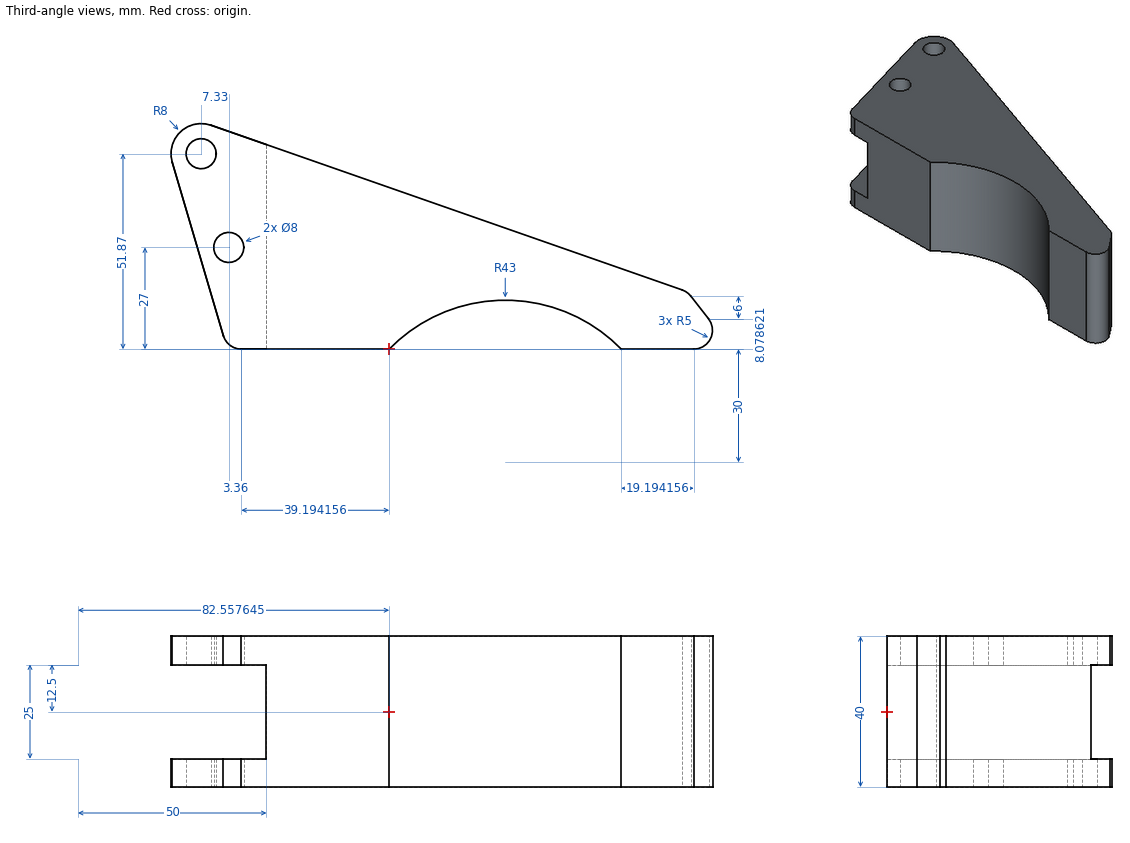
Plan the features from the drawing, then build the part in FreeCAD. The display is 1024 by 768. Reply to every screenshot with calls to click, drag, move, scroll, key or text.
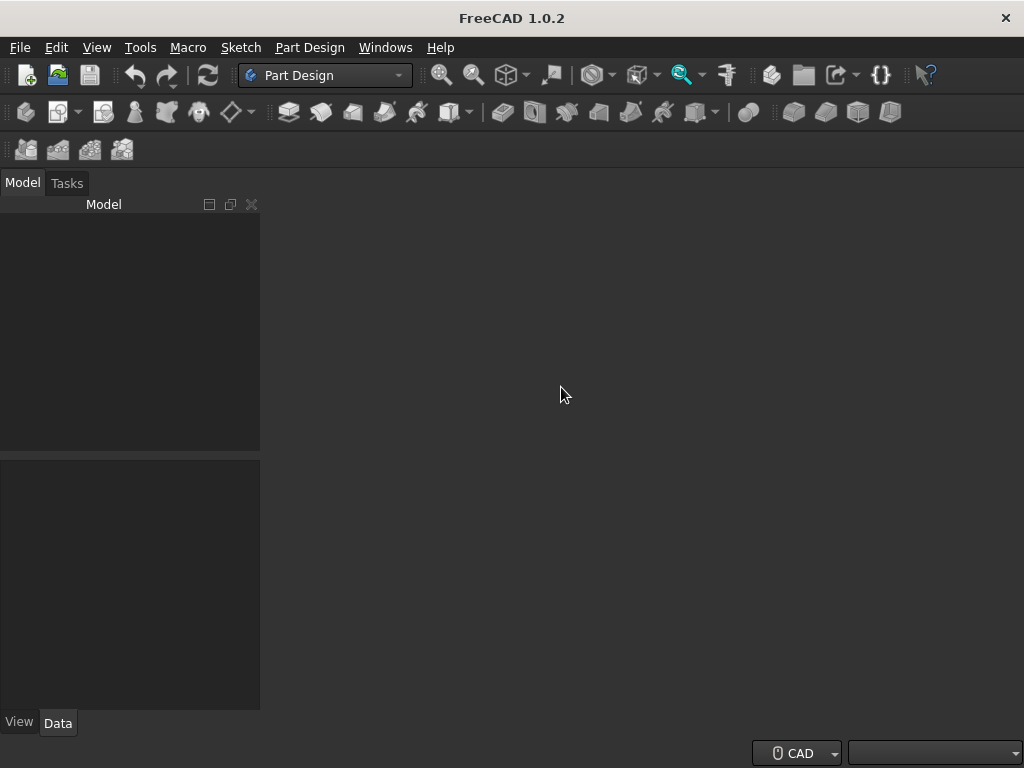
click(26, 76)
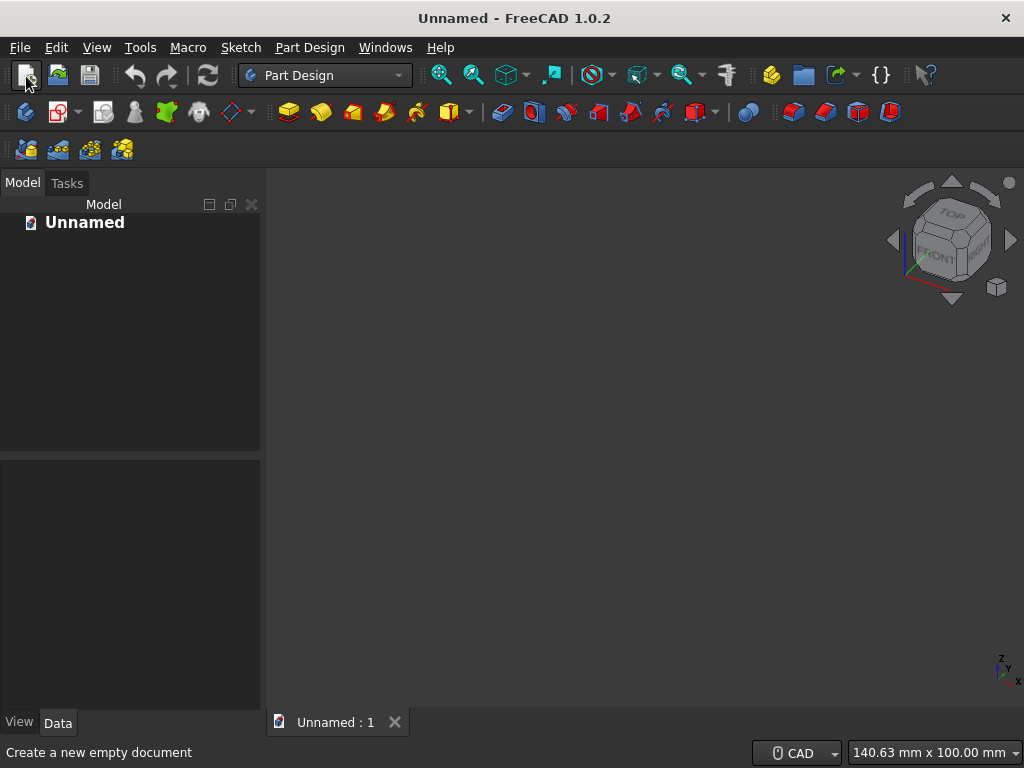
click(58, 112)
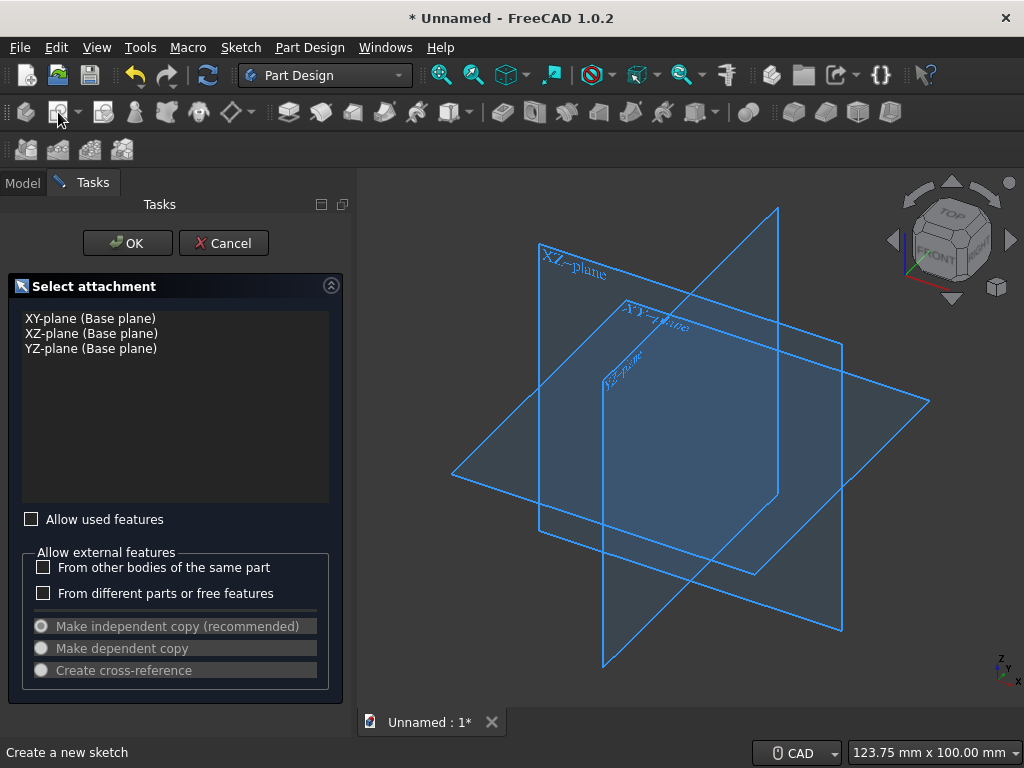
click(82, 318)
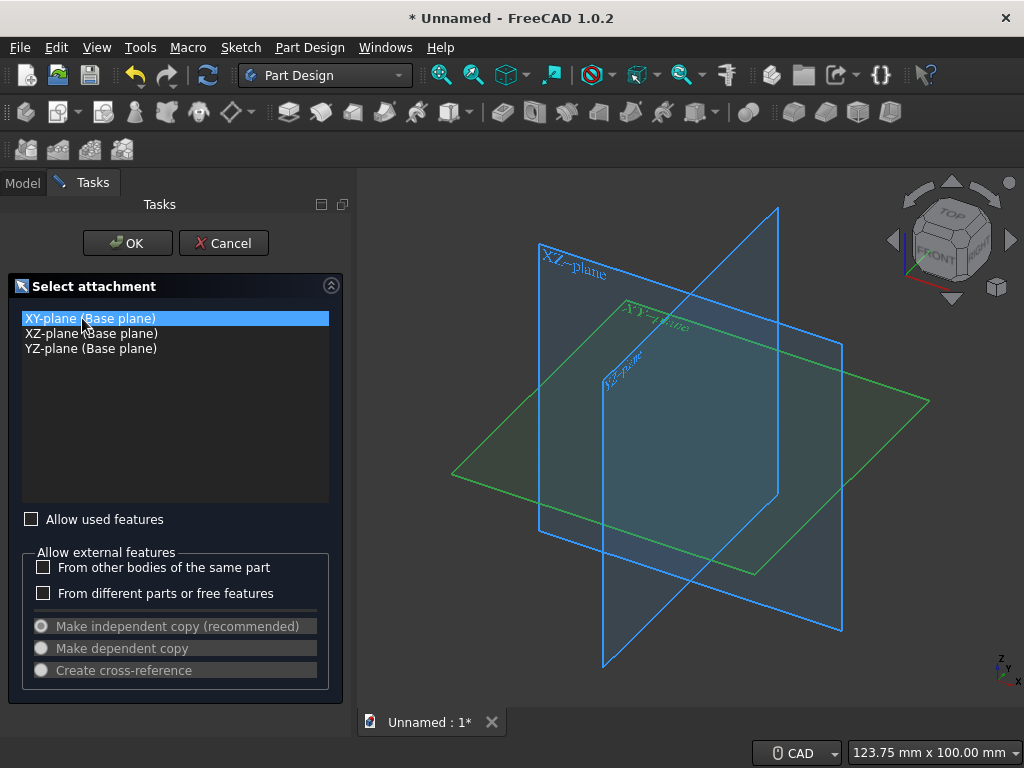
click(128, 243)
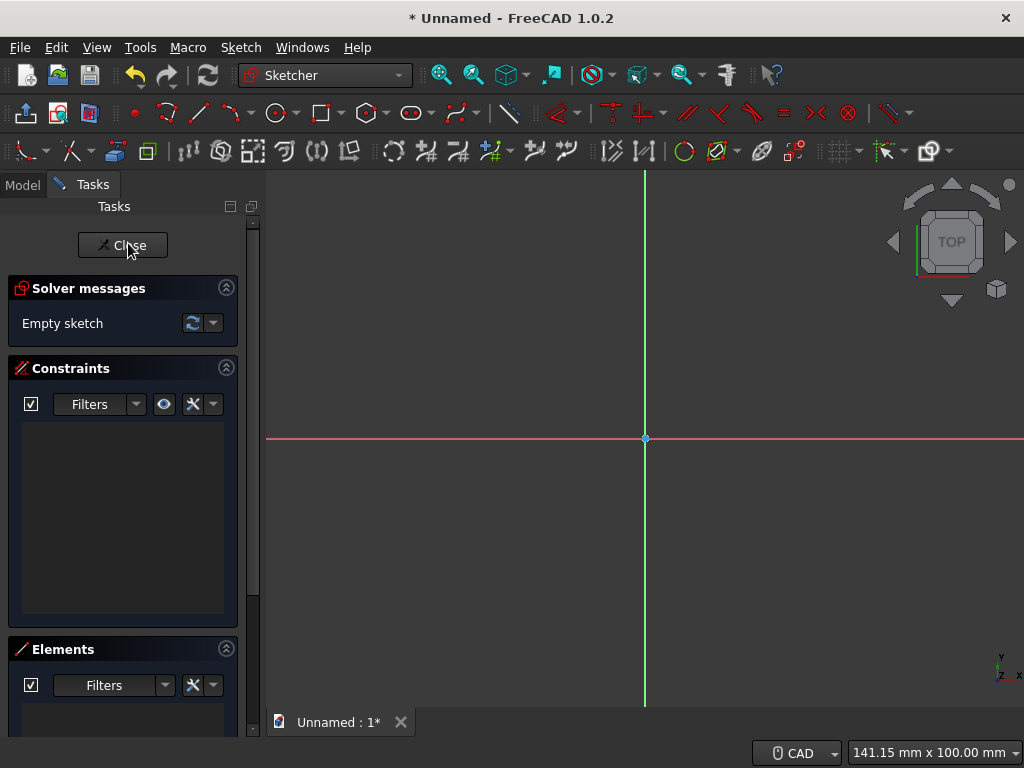
scroll(403, 633, down, 3)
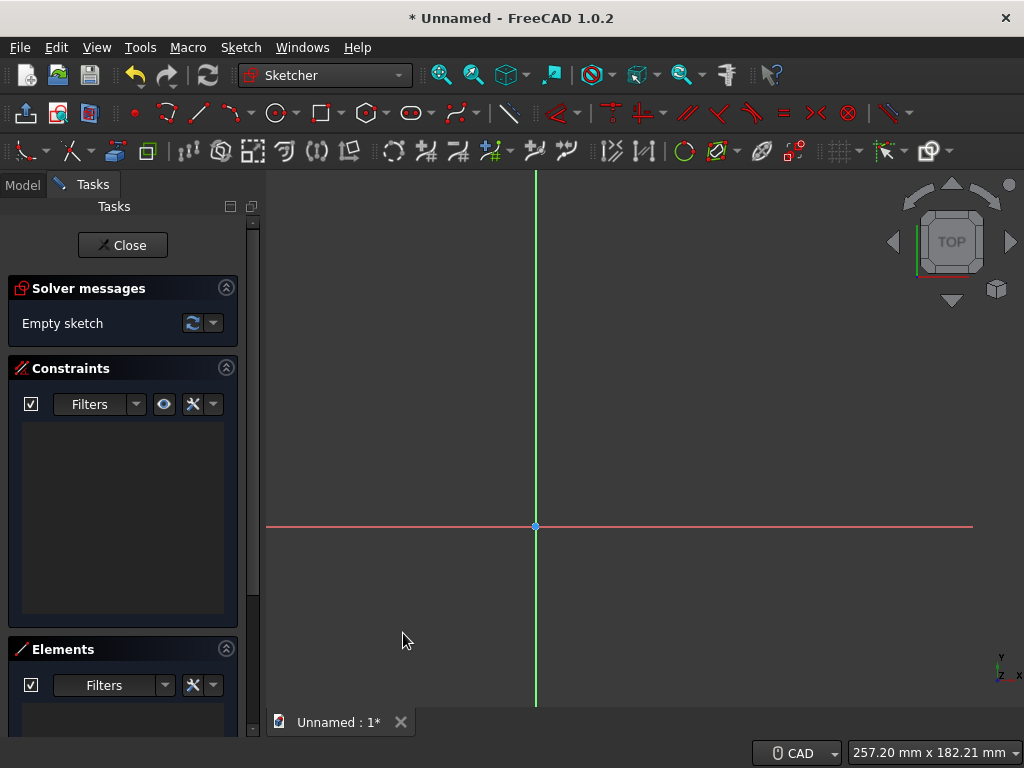
click(200, 114)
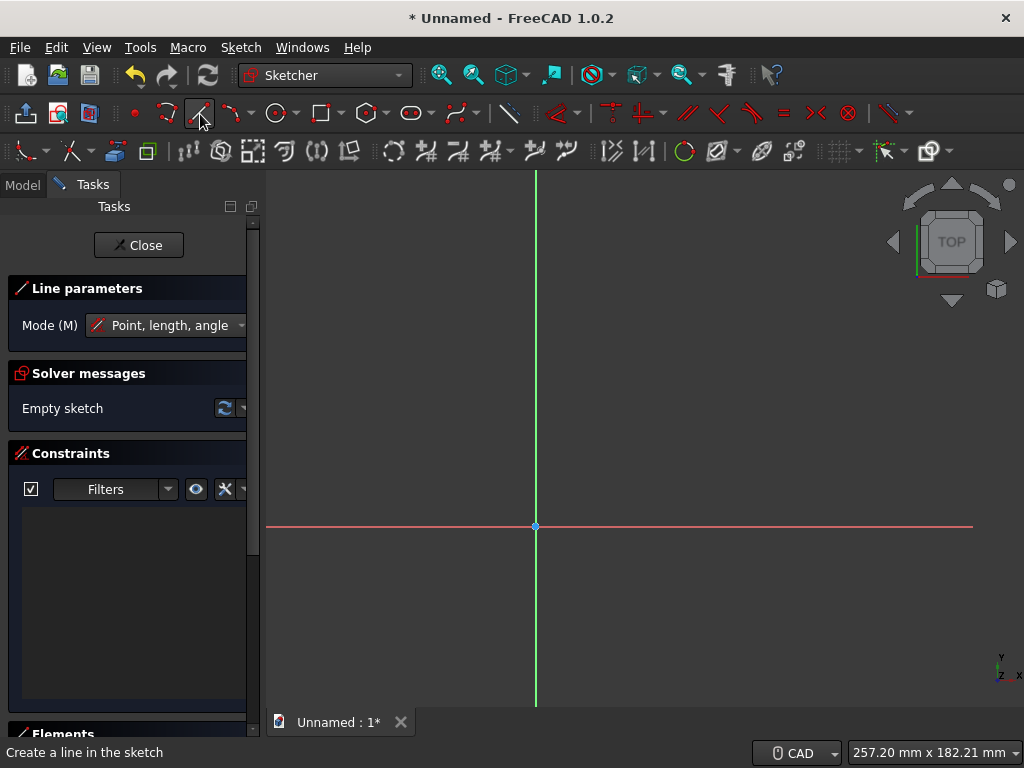
click(420, 527)
click(536, 527)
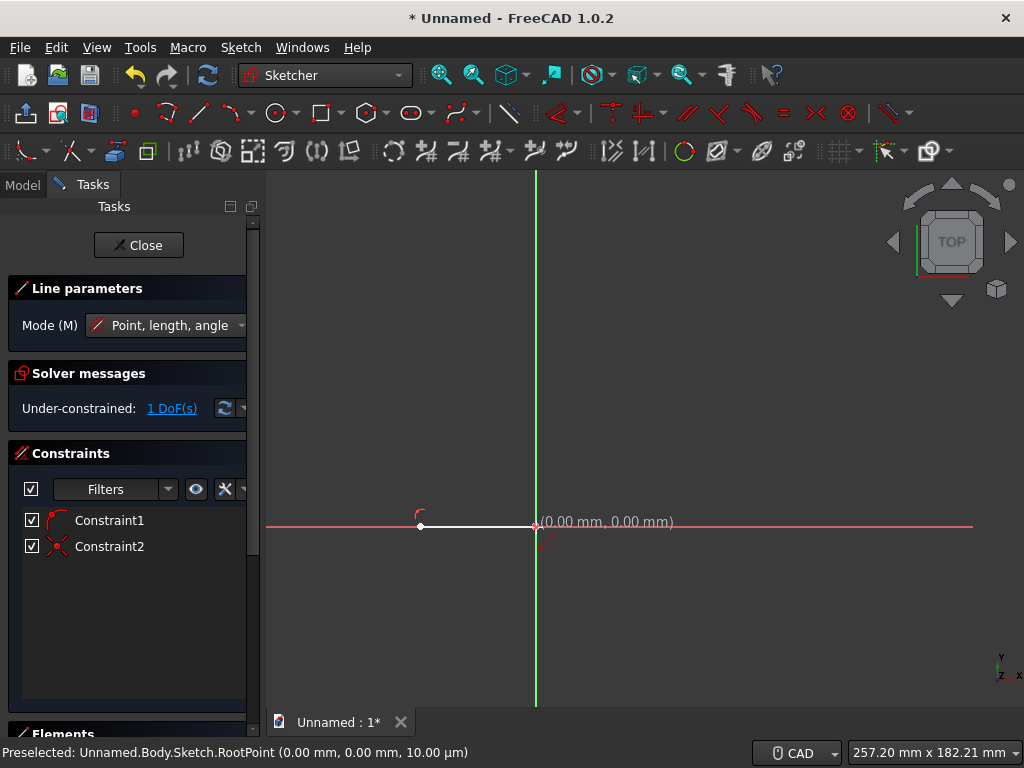
click(717, 527)
click(774, 518)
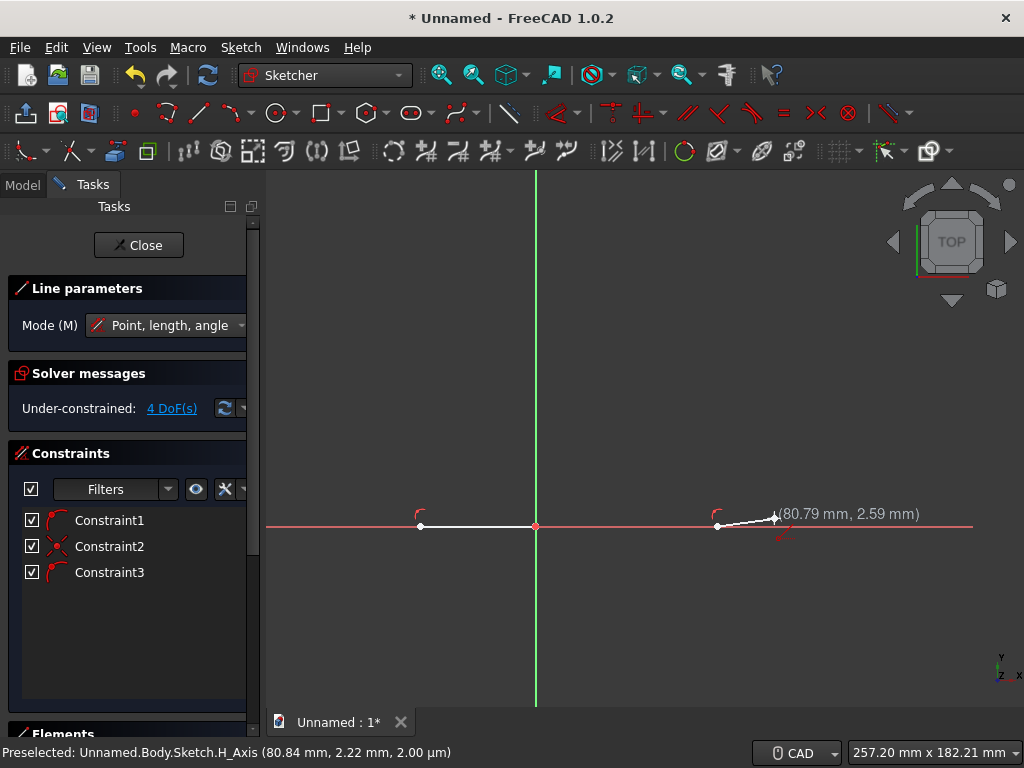
click(786, 503)
click(772, 485)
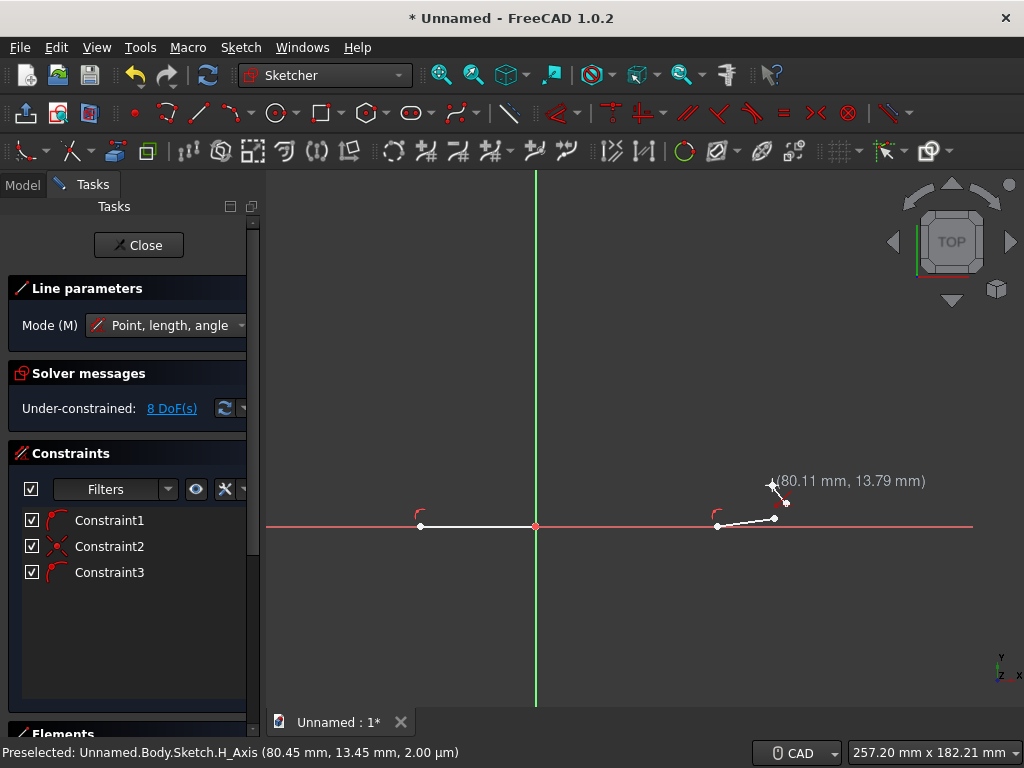
scroll(765, 480, up, 4)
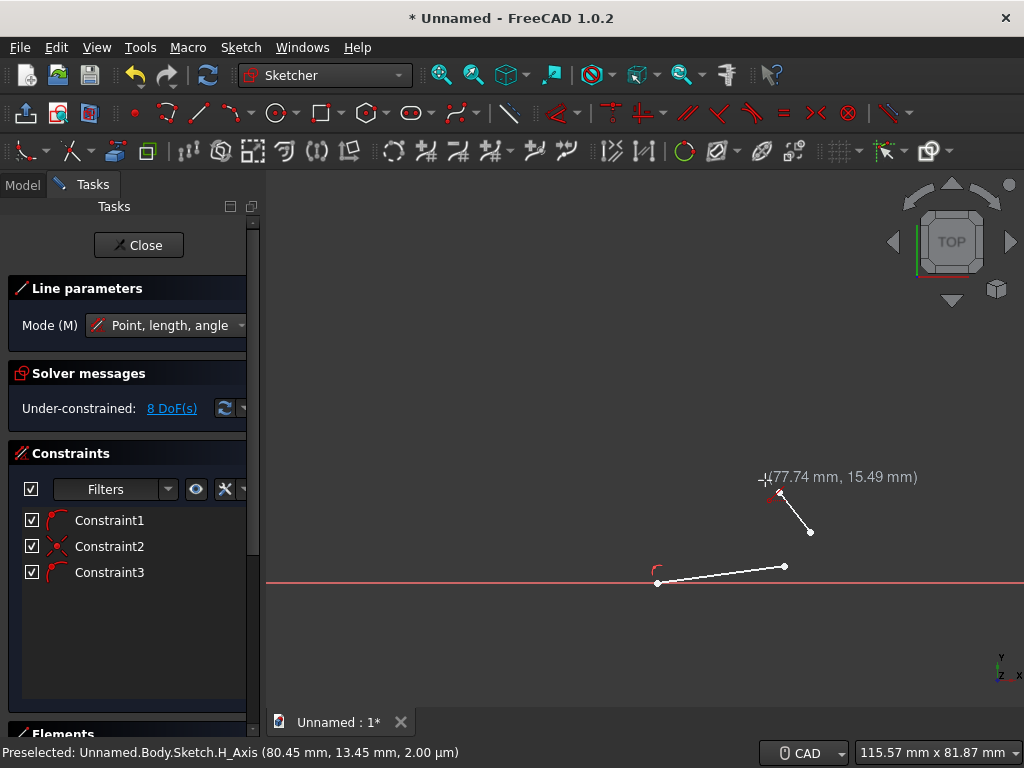
click(764, 480)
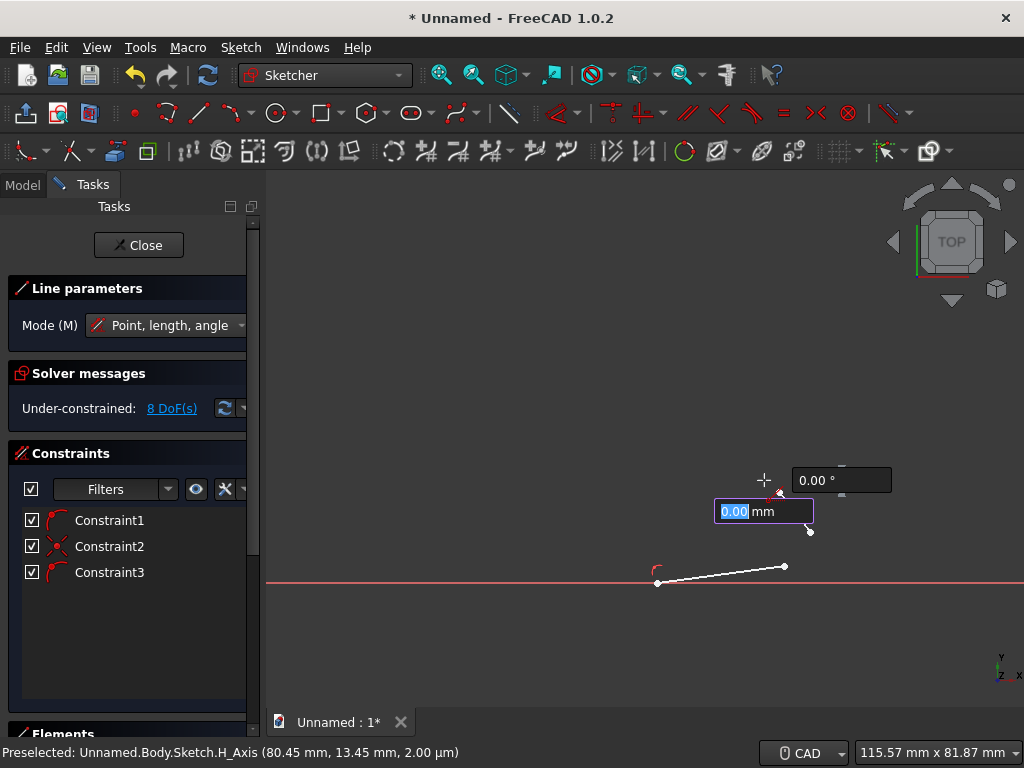
scroll(765, 480, down, 4)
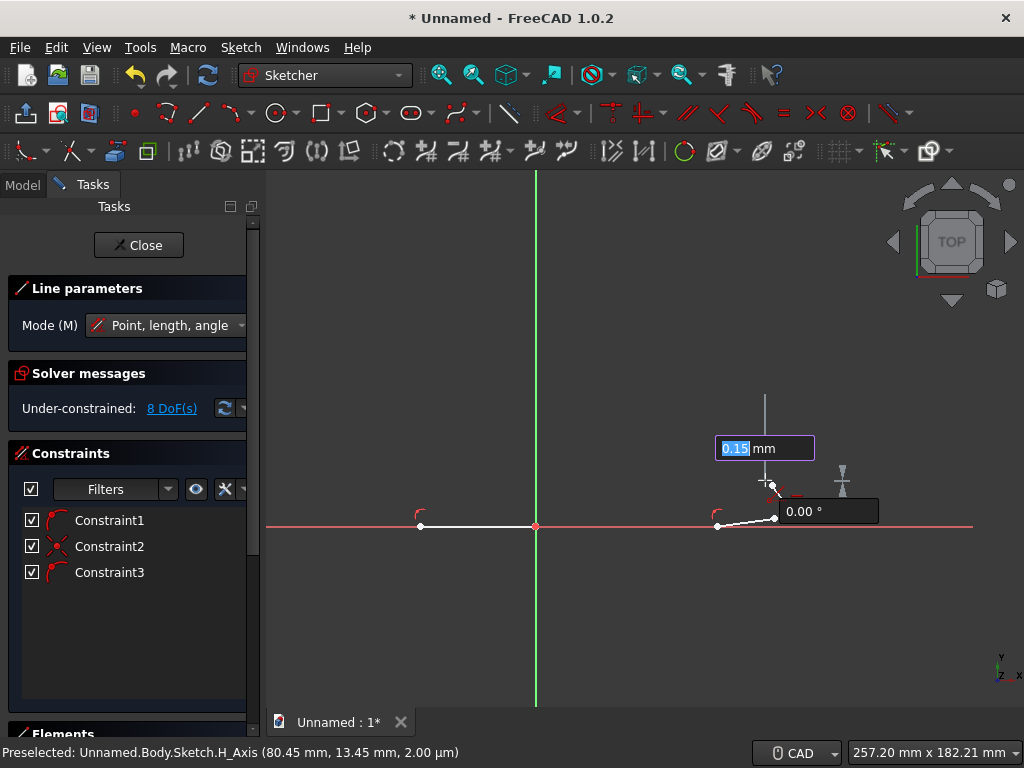
click(397, 352)